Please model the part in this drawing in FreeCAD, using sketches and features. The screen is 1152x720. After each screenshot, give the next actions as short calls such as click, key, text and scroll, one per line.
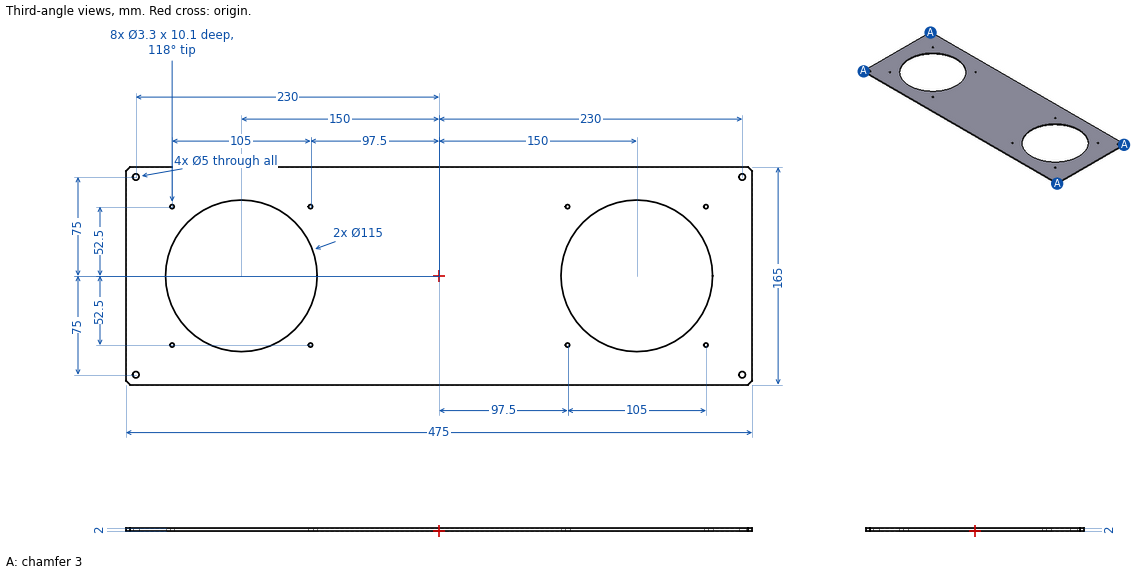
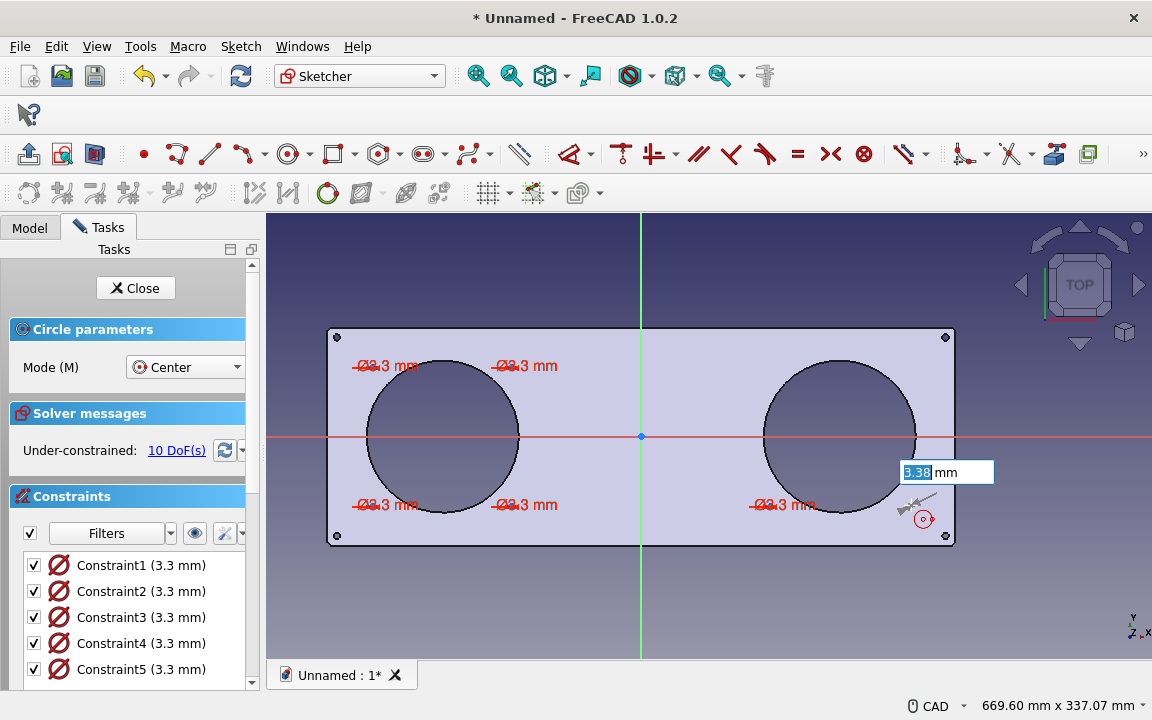
text(3.3)
key(Return)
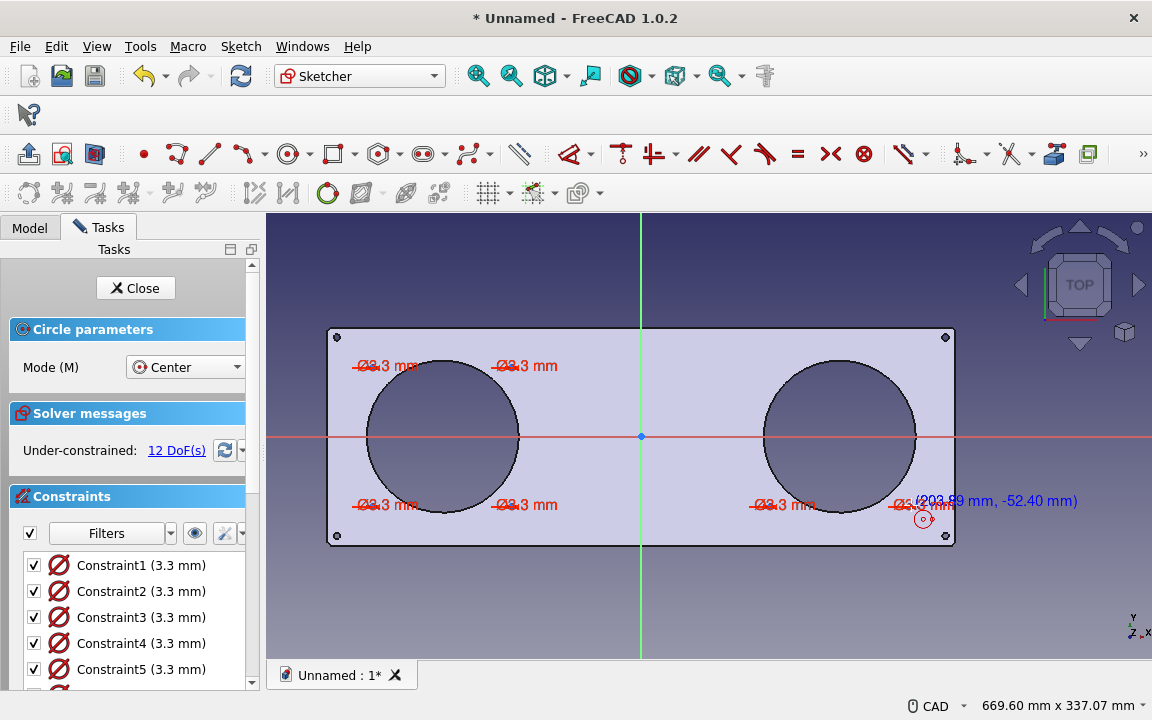
scroll(909, 367, up, 12)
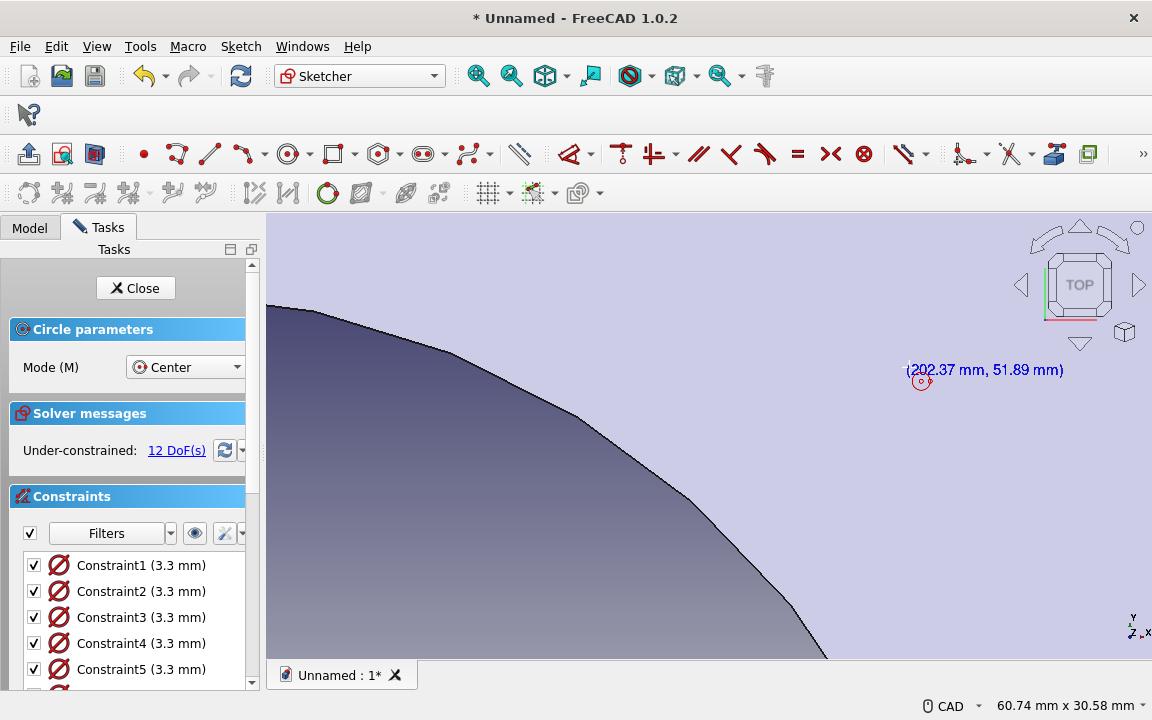
scroll(909, 367, down, 12)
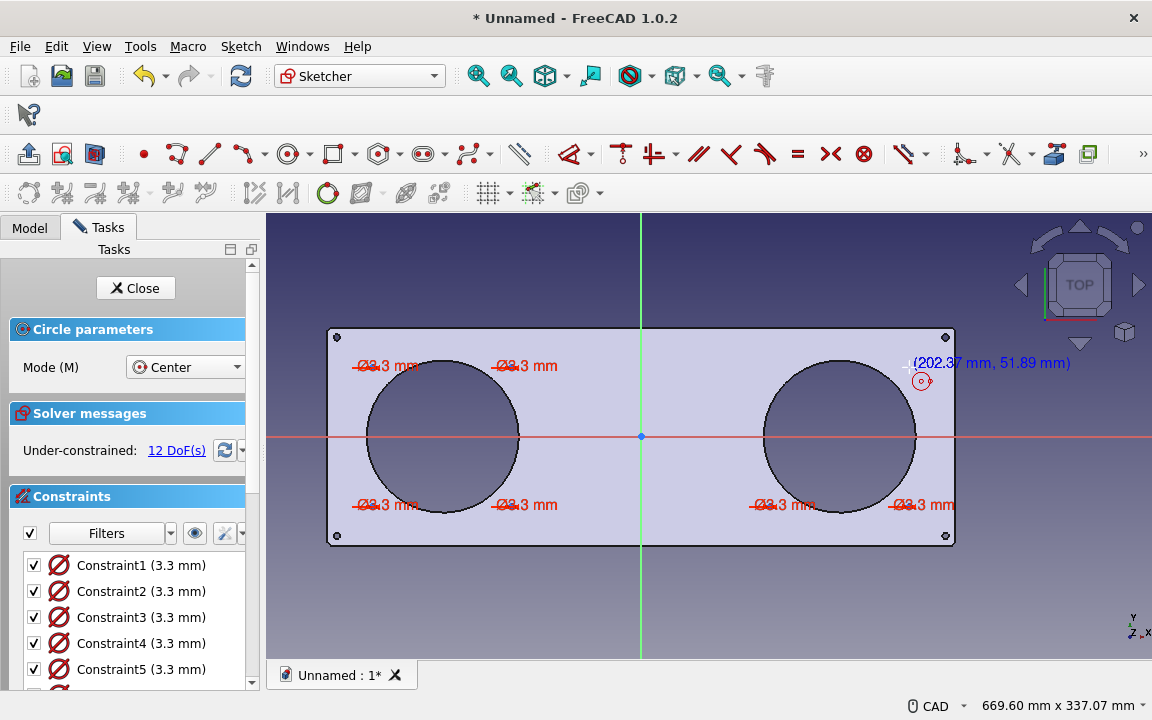
click(909, 367)
move(911, 366)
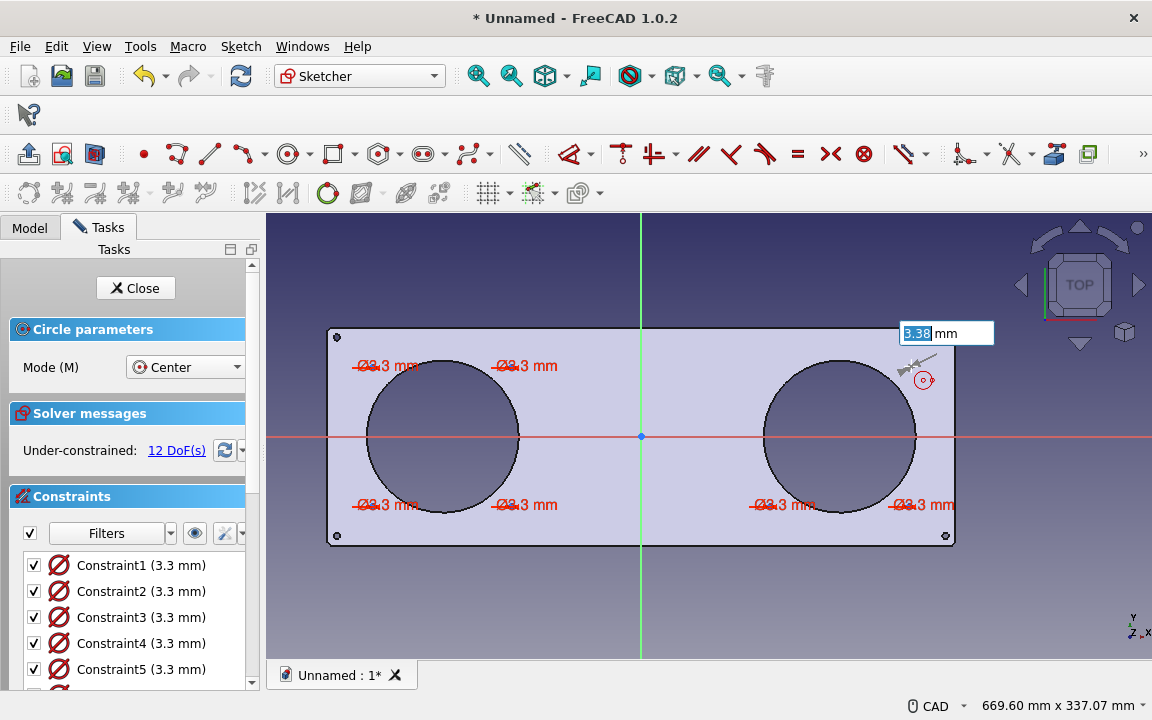
text(3.3)
key(Return)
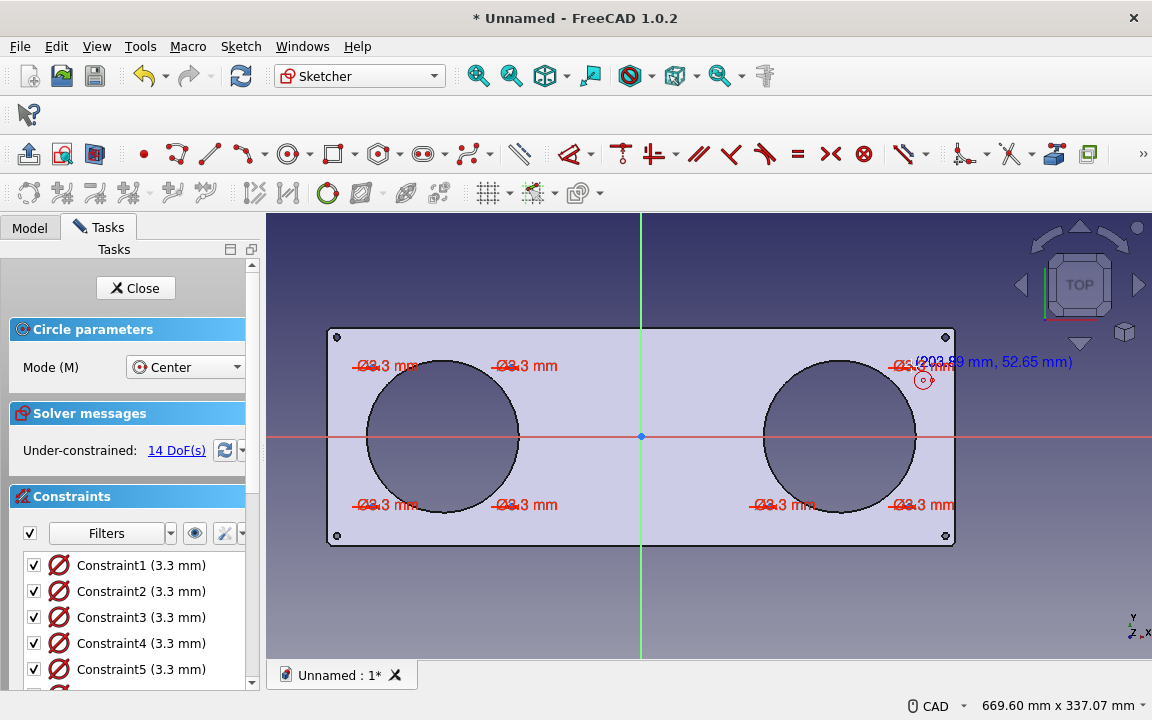
scroll(770, 367, up, 12)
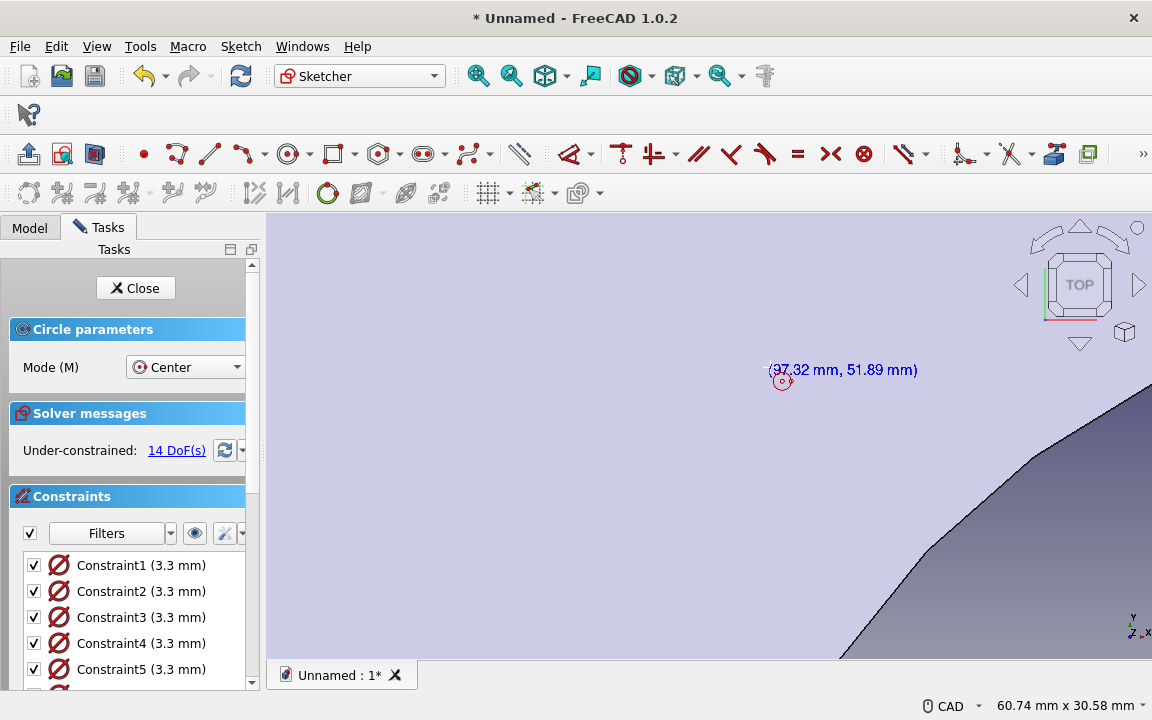
scroll(770, 367, down, 12)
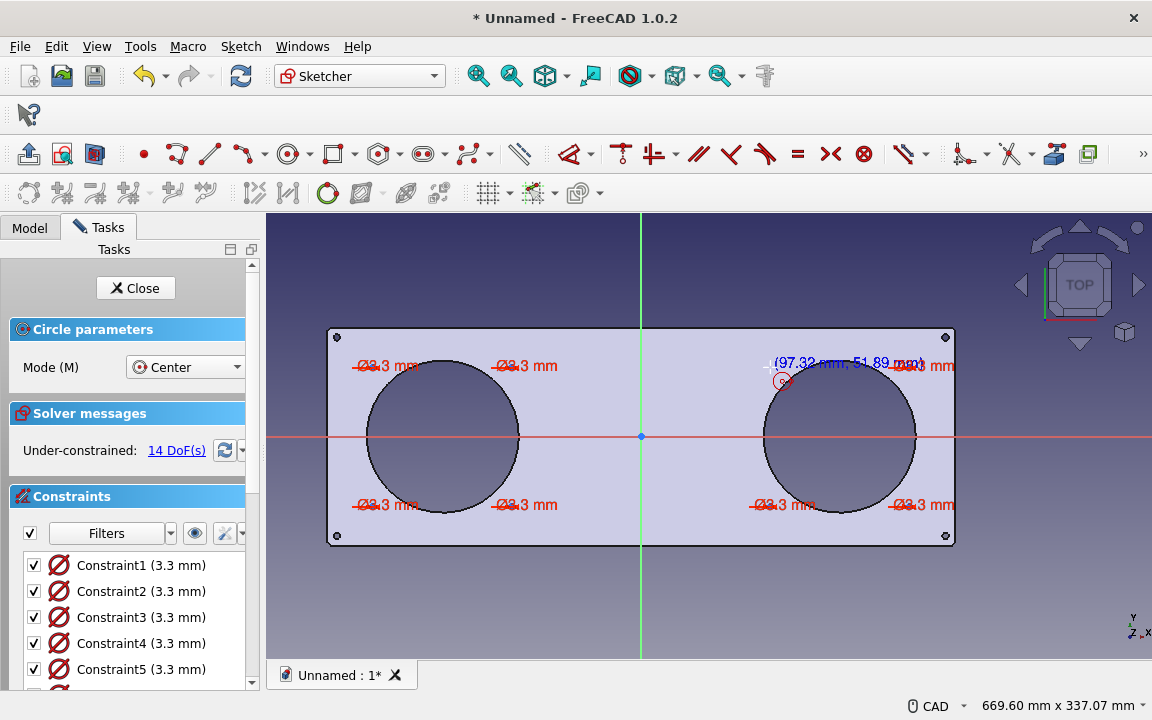
click(770, 367)
move(772, 366)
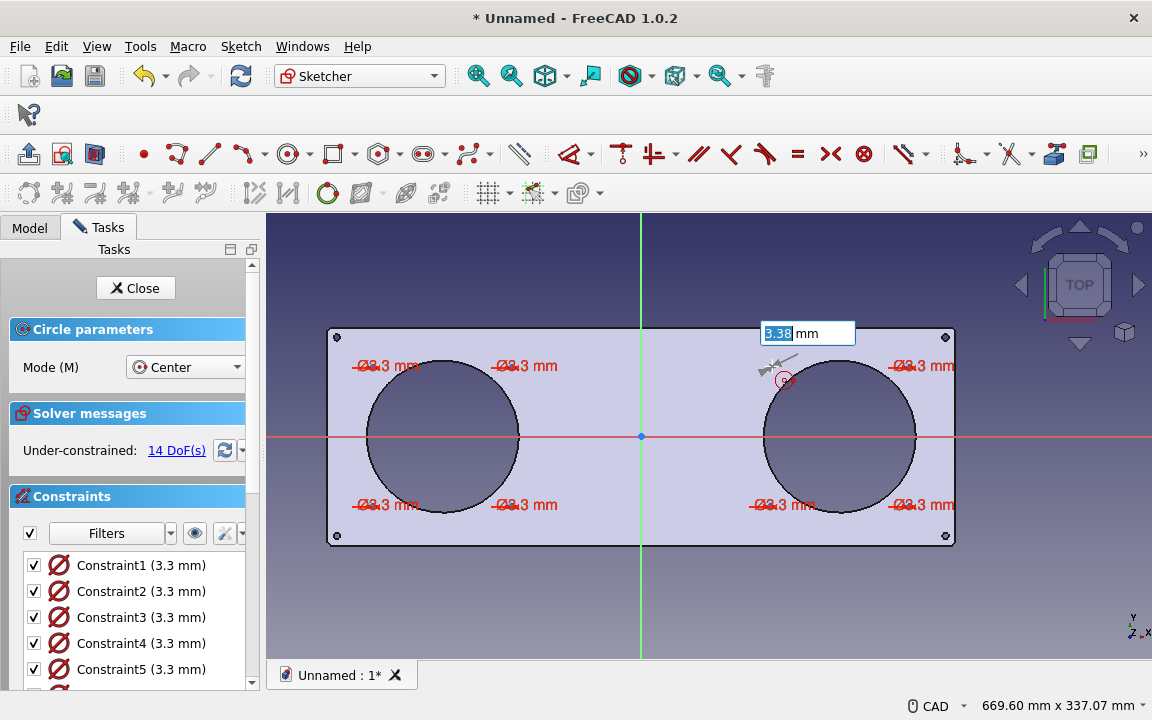
text(3.3)
key(Return)
key(Escape)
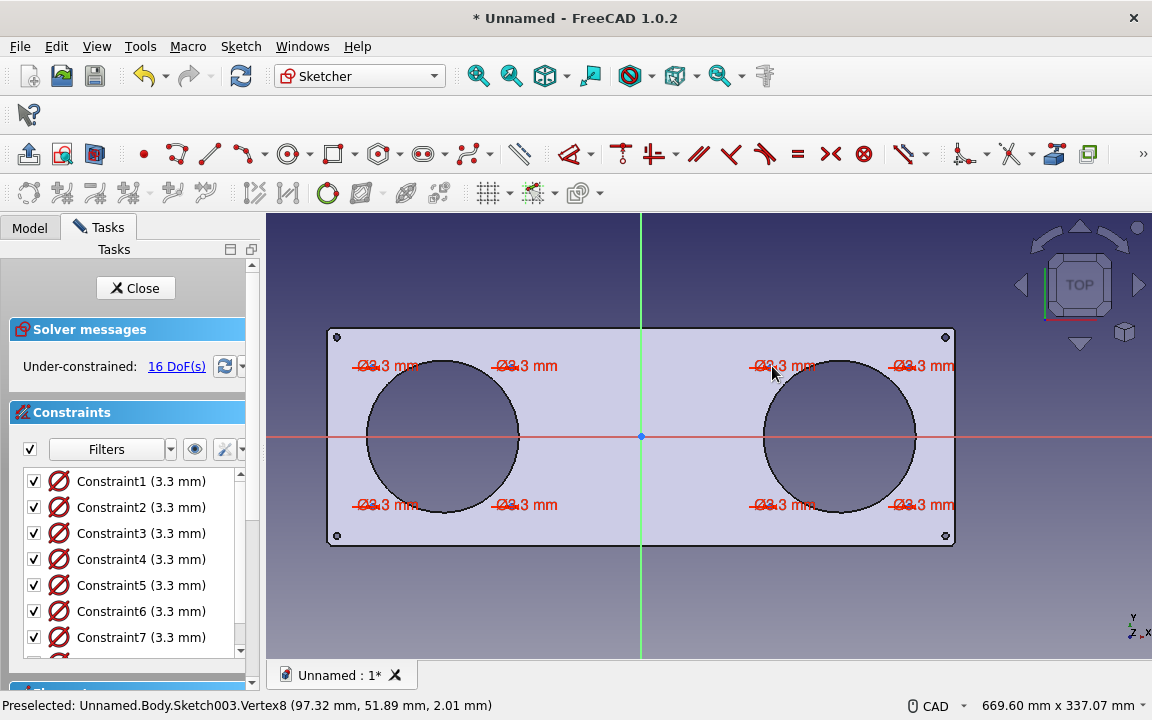
click(373, 368)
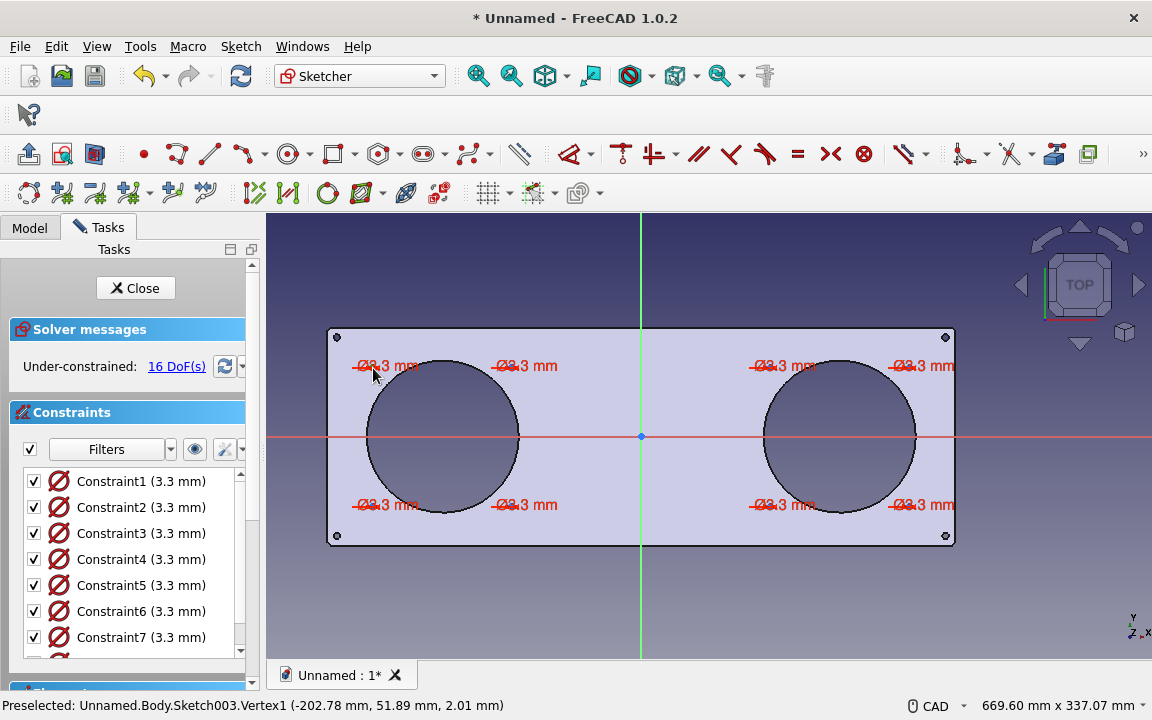
click(512, 368)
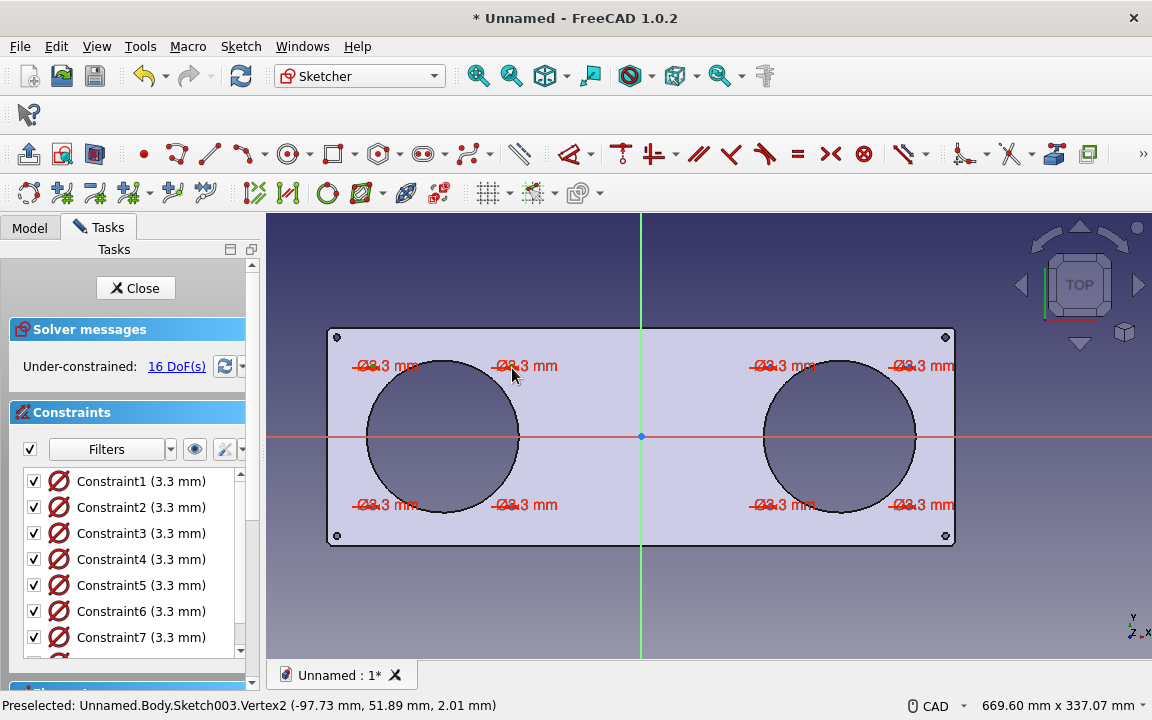
key(h)